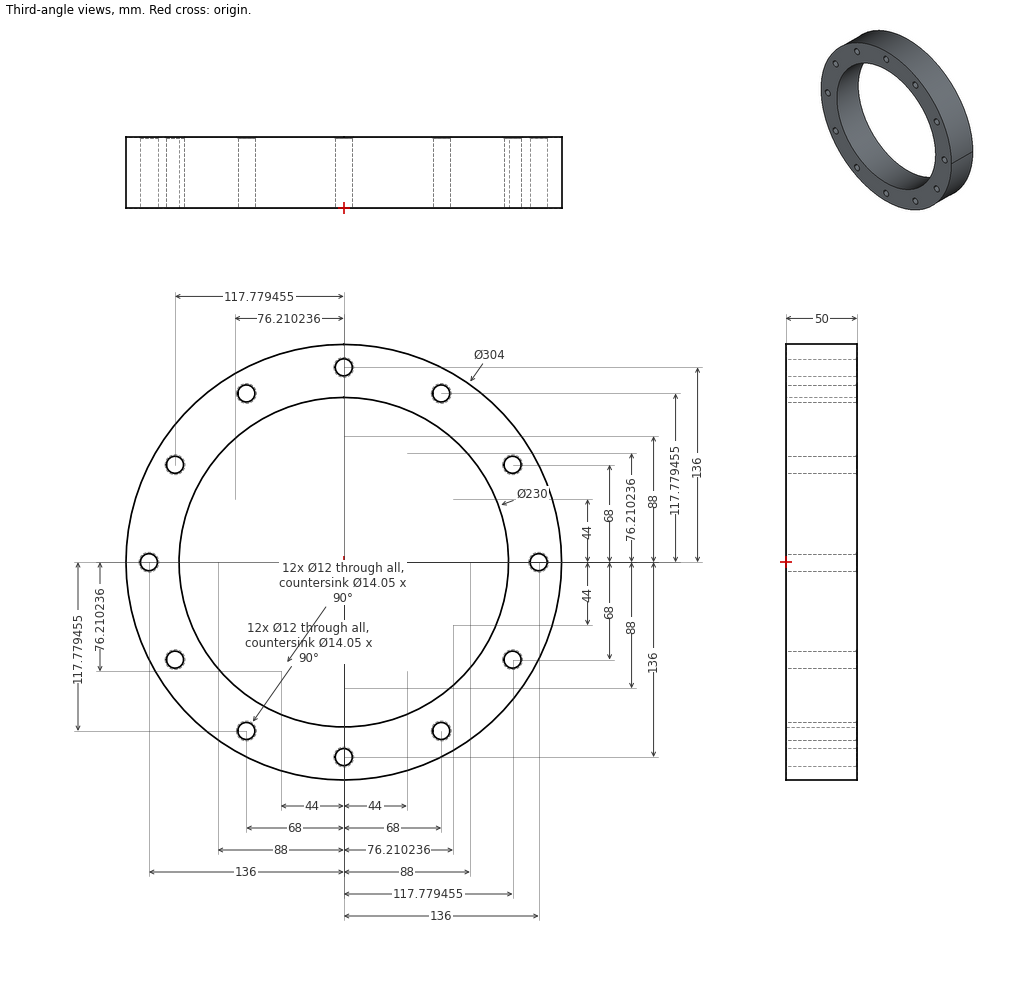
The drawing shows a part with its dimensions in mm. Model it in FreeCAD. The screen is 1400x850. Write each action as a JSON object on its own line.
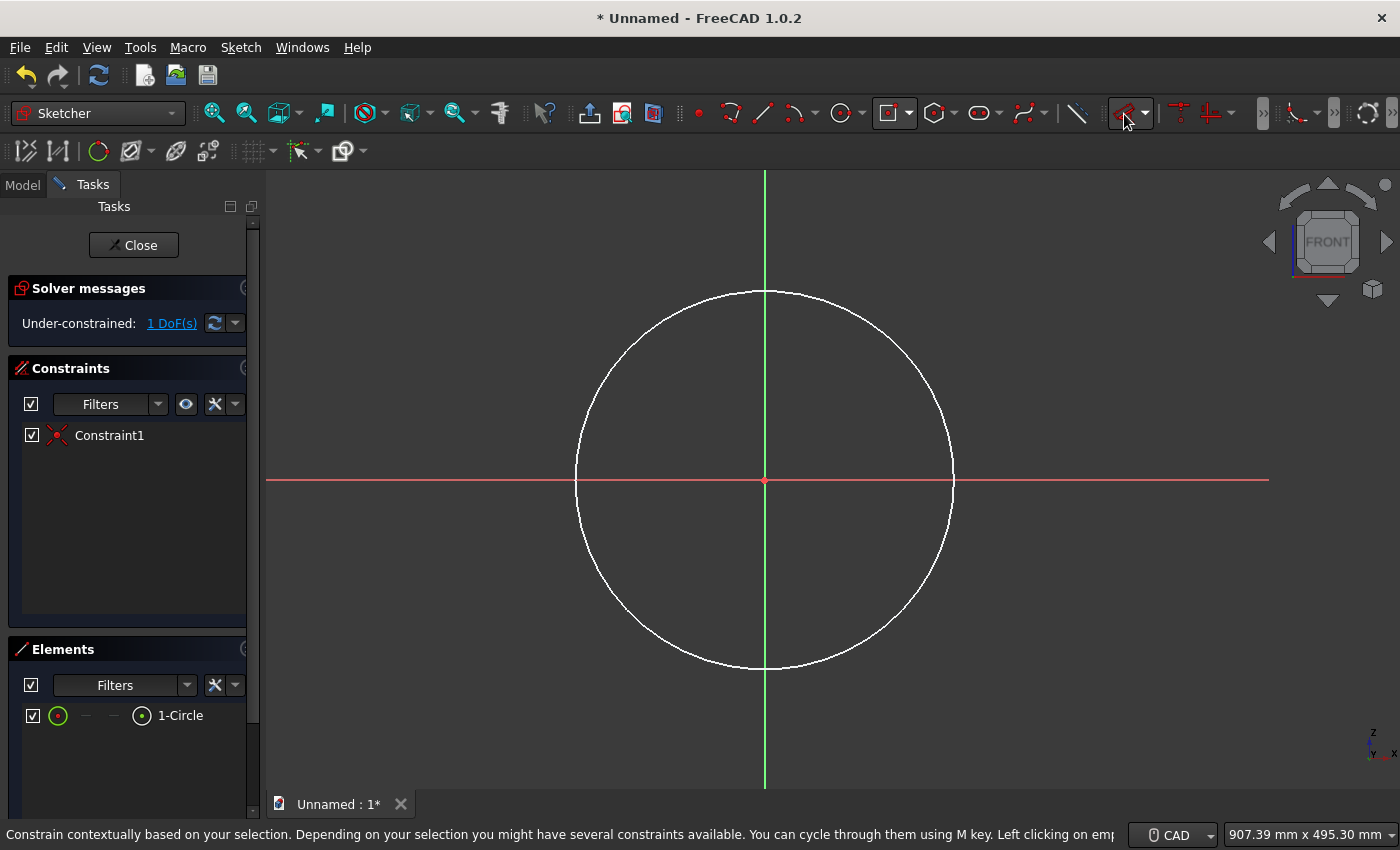
{"action": "left_click", "coordinate": [898, 346]}
{"action": "left_click", "coordinate": [921, 323]}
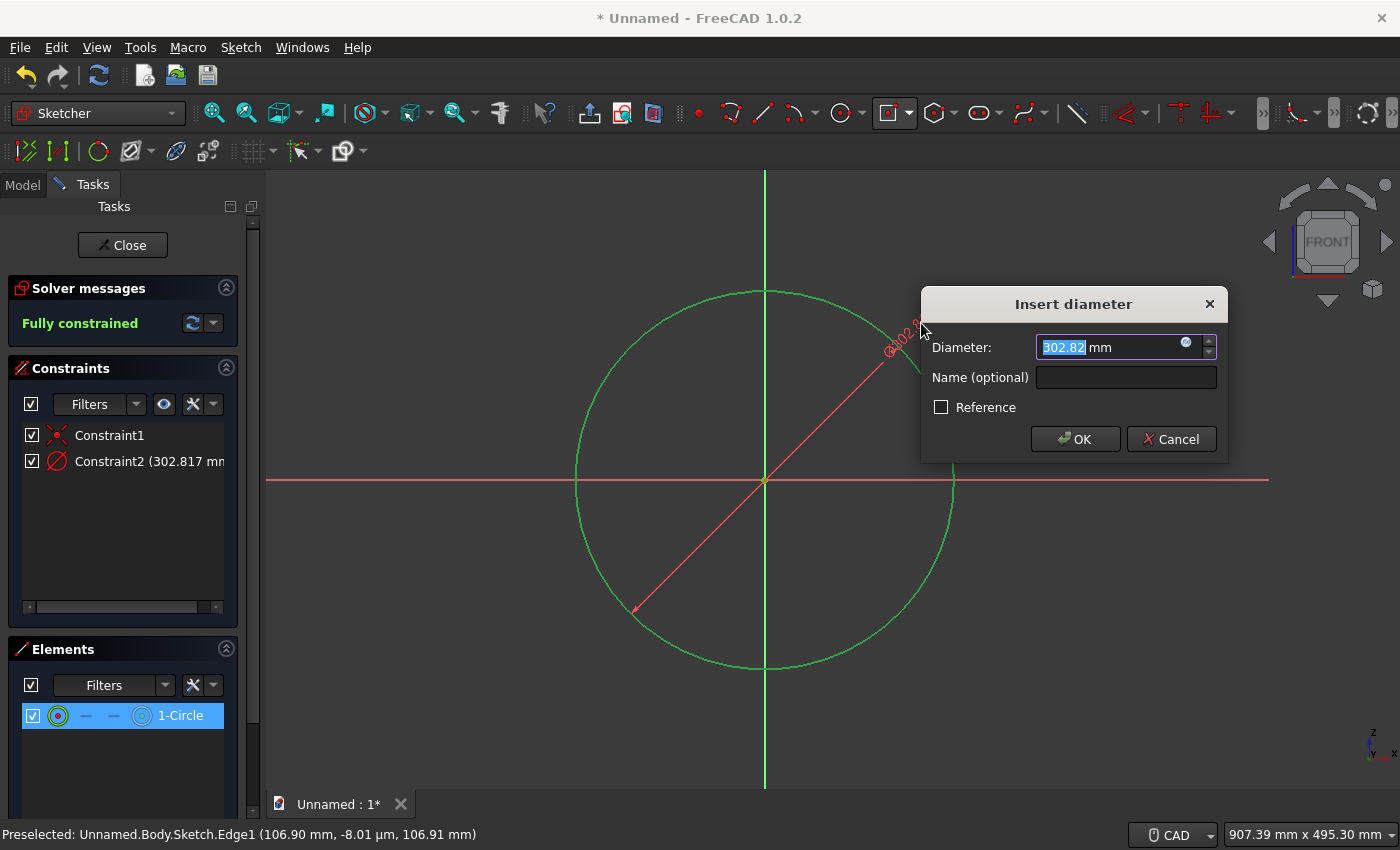
{"action": "type", "text": "304"}
{"action": "key", "text": "Return"}
{"action": "key", "text": "Escape"}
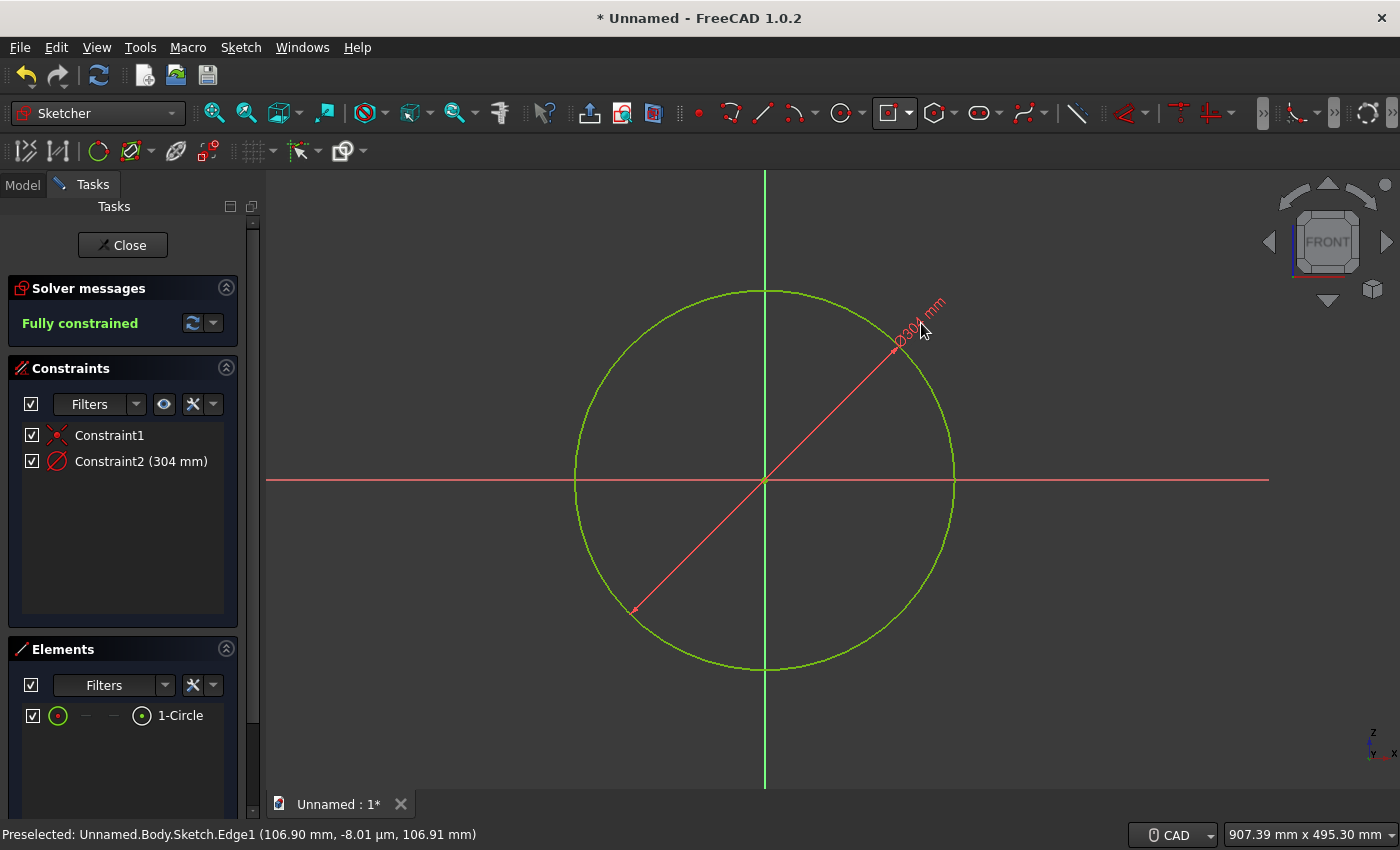
{"action": "left_click", "coordinate": [123, 245]}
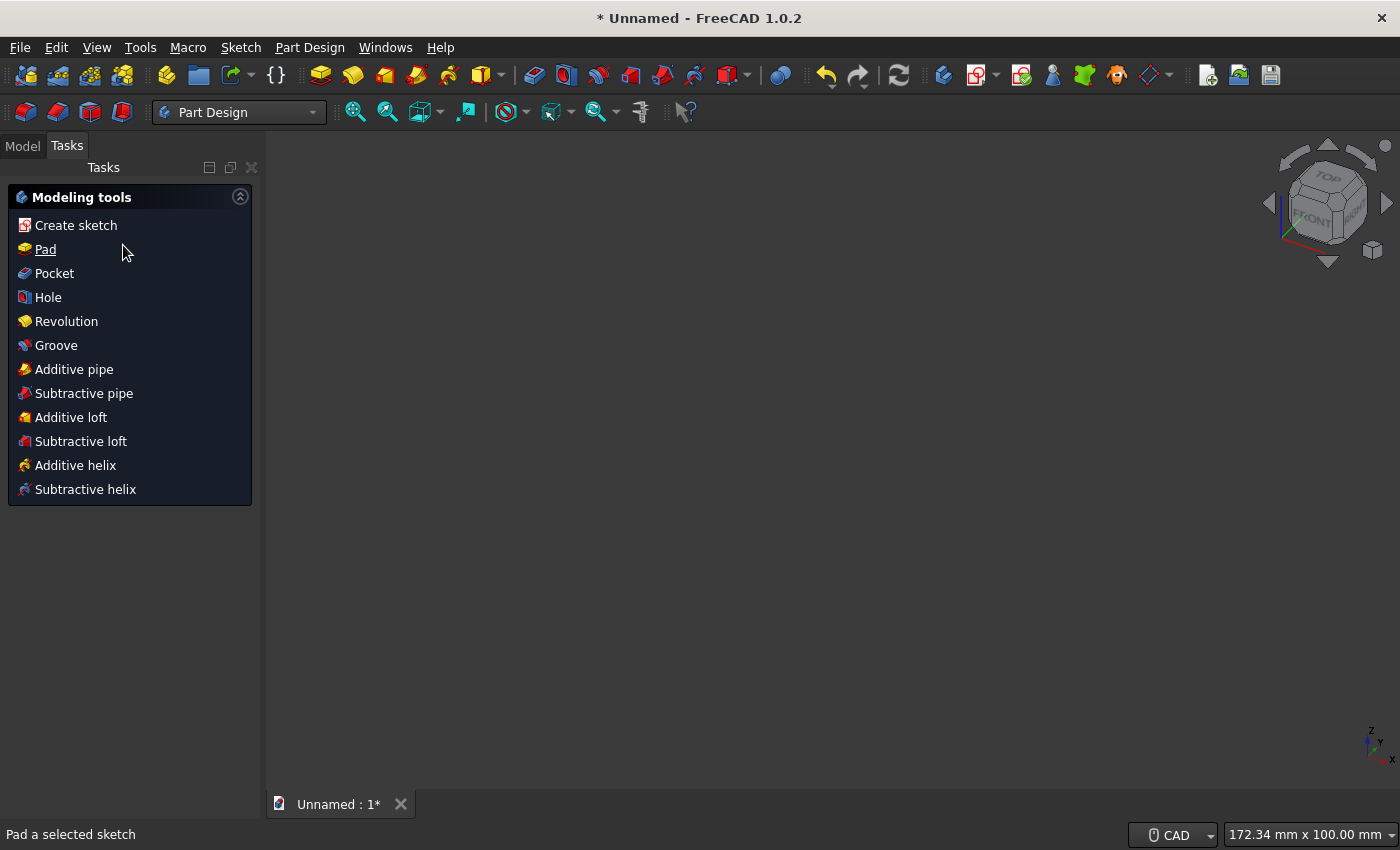
{"action": "left_click", "coordinate": [322, 76]}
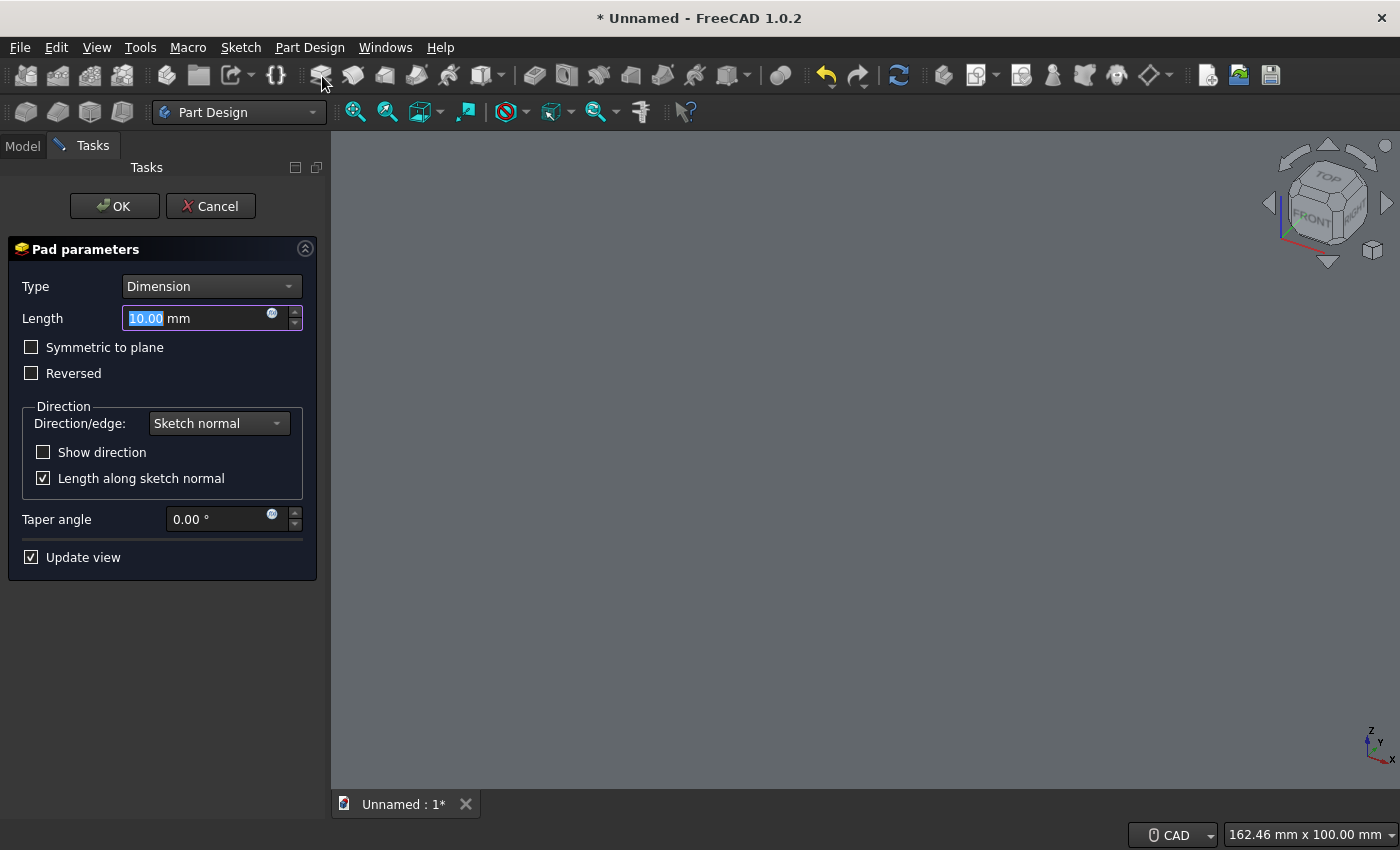
{"action": "type", "text": "50"}
{"action": "key", "text": "Tab"}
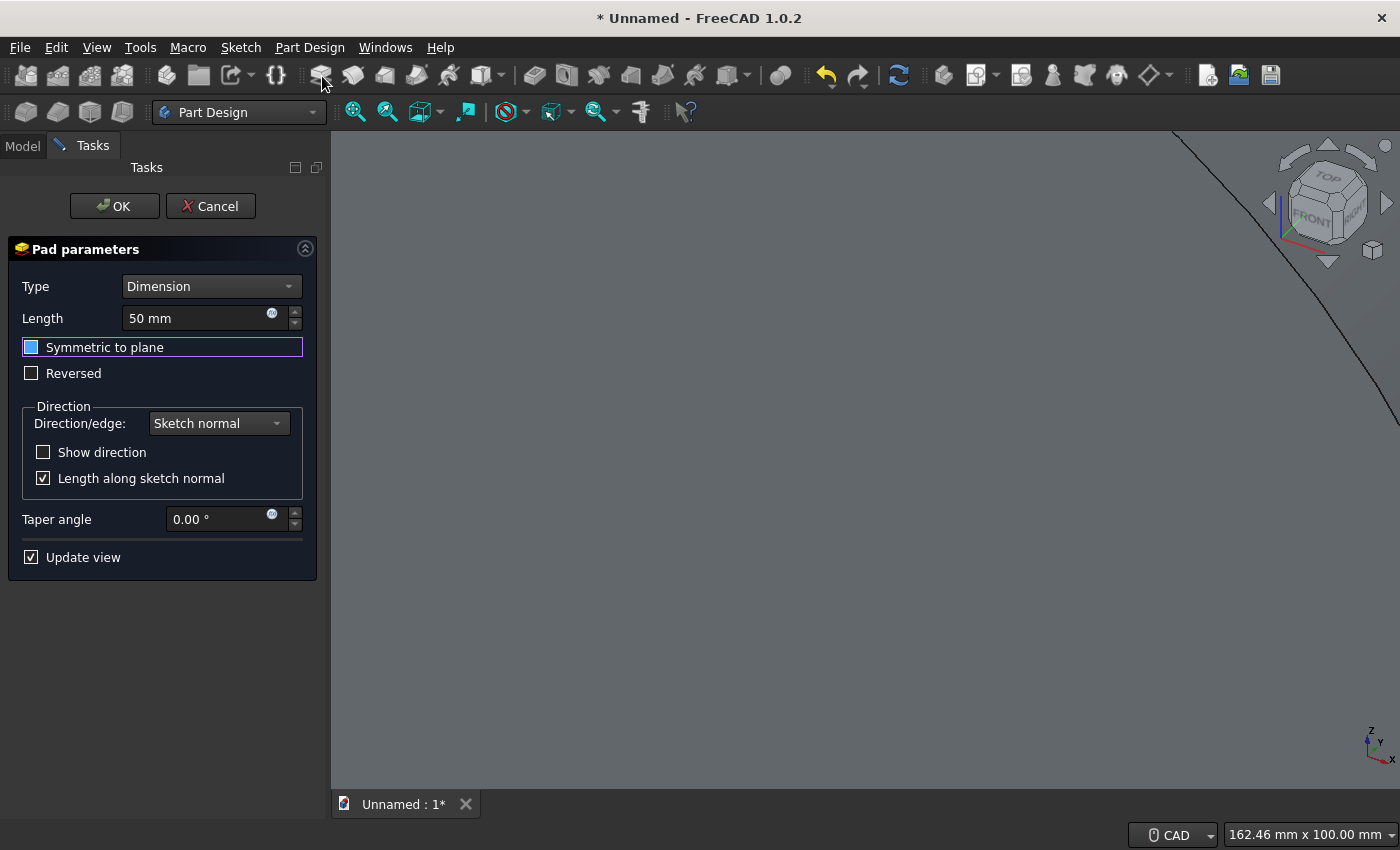
{"action": "left_click", "coordinate": [30, 373]}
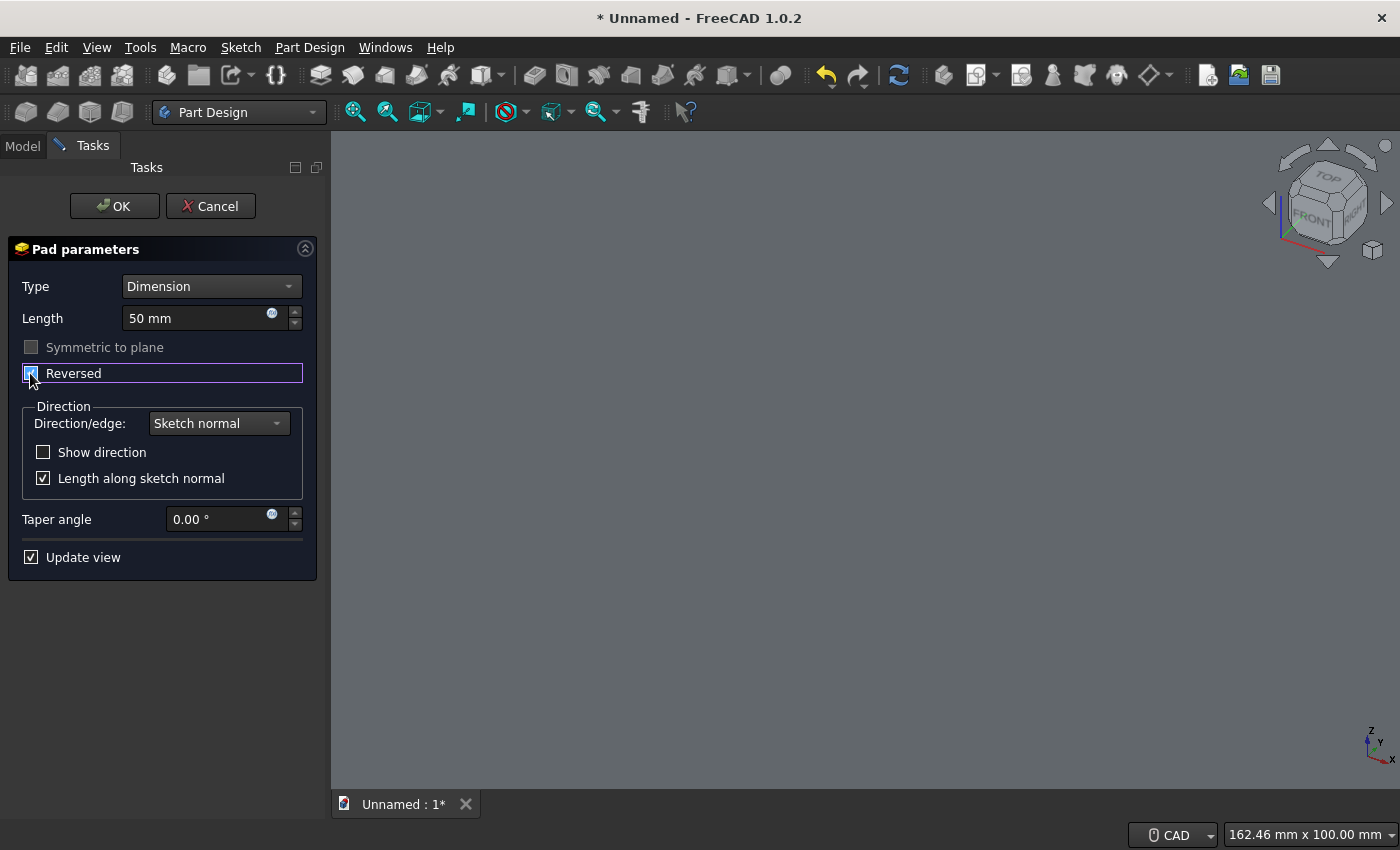
{"action": "left_click", "coordinate": [115, 206]}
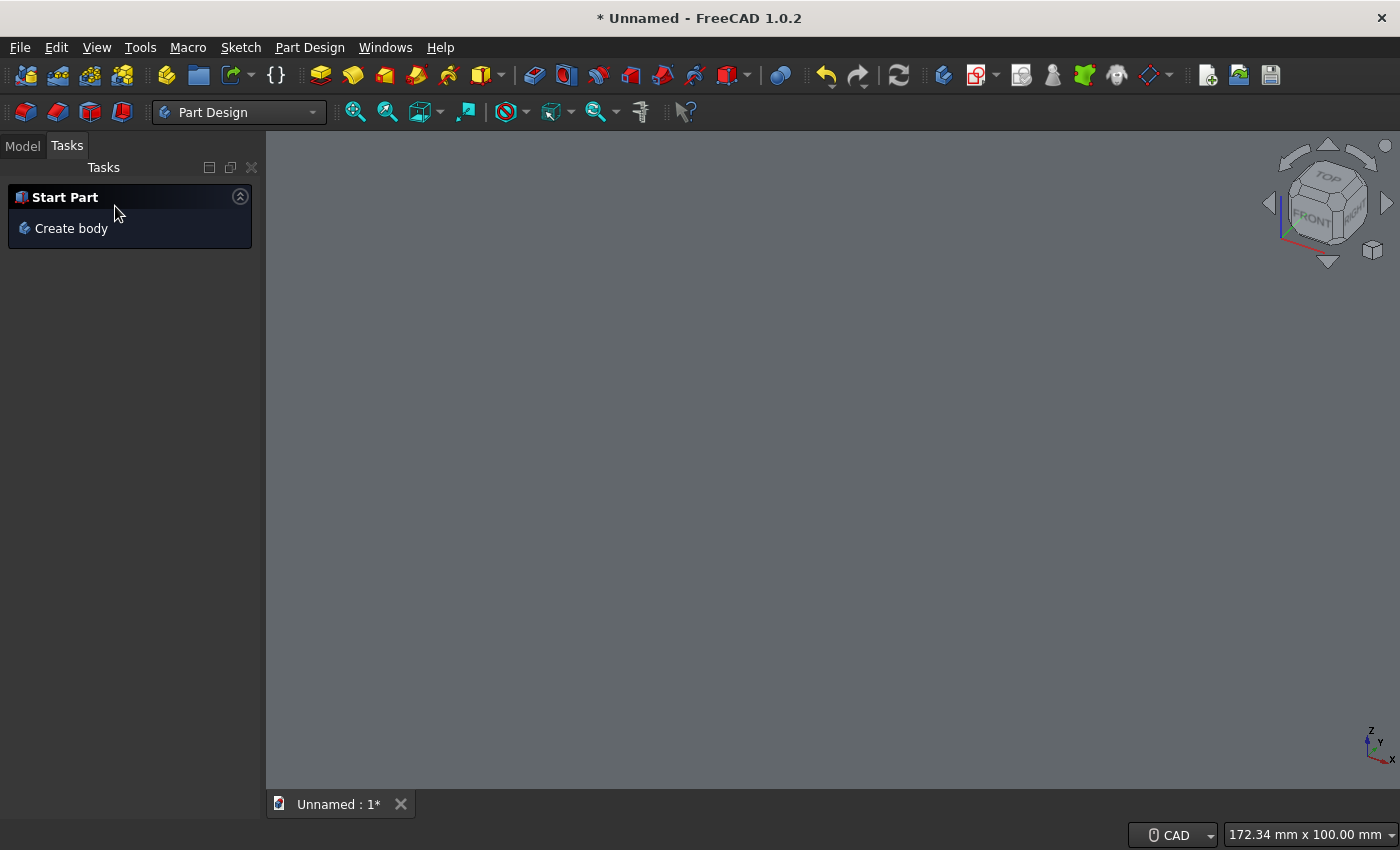
{"action": "key", "text": "v f"}